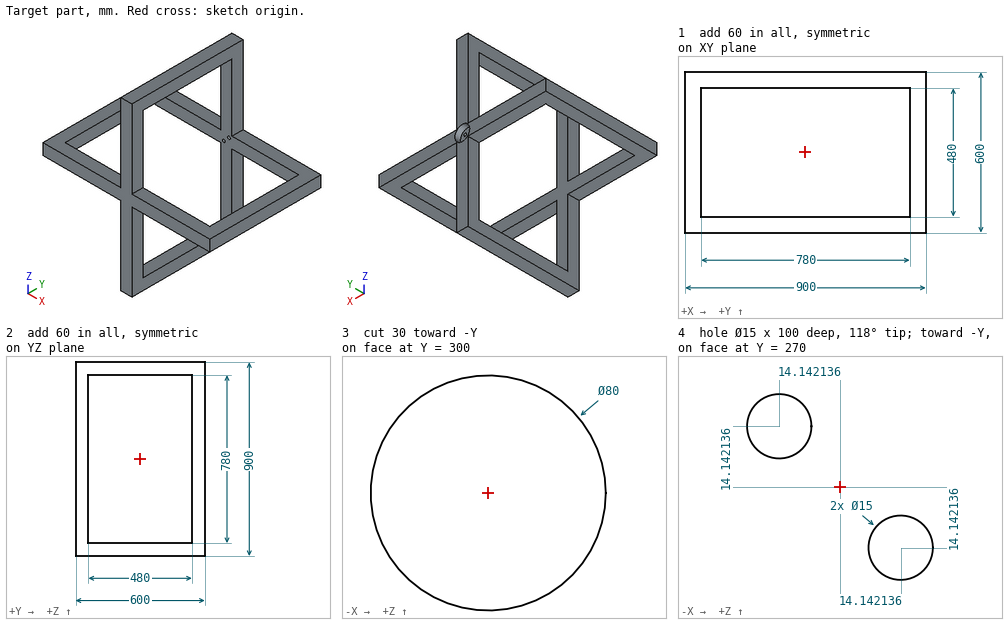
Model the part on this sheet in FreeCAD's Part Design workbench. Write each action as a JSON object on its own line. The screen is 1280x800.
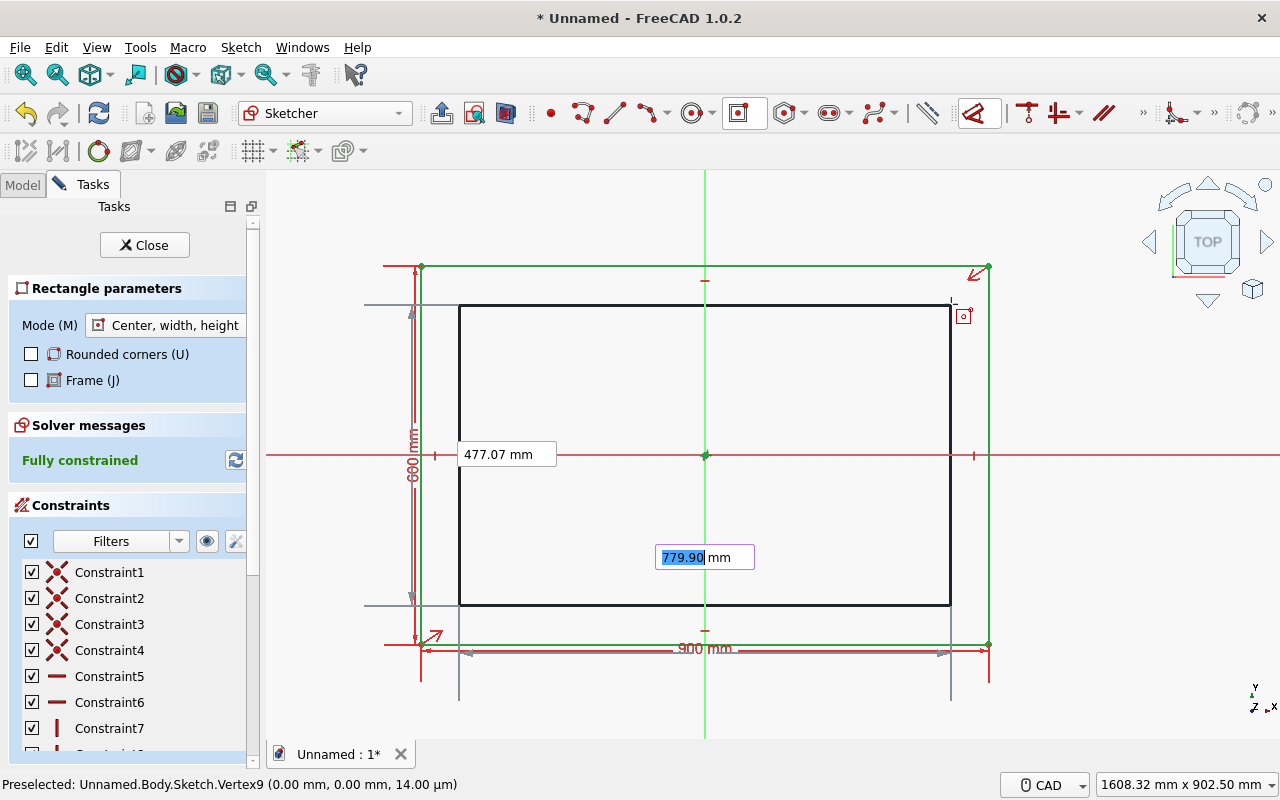
{"action": "type", "text": "780"}
{"action": "key", "text": "Tab"}
{"action": "type", "text": "480"}
{"action": "key", "text": "Return"}
{"action": "key", "text": "Escape"}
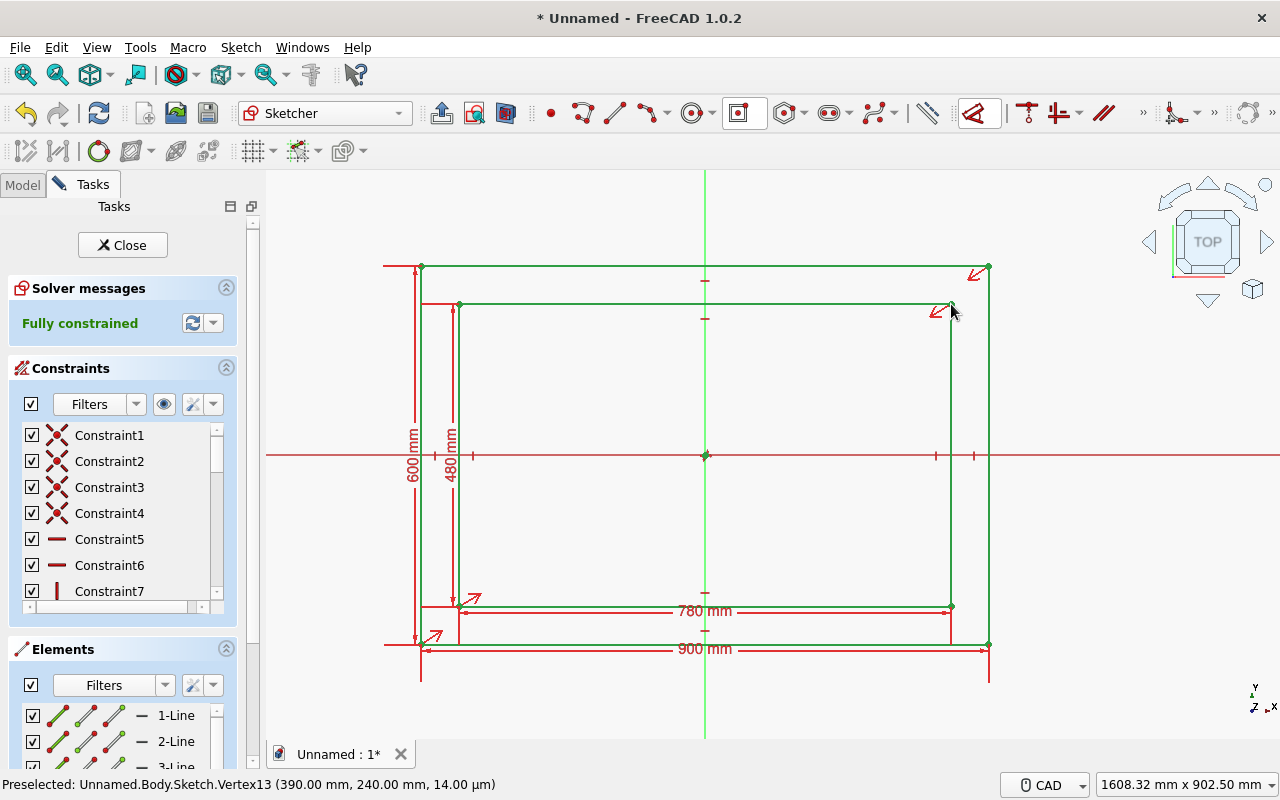
{"action": "left_click", "coordinate": [123, 245]}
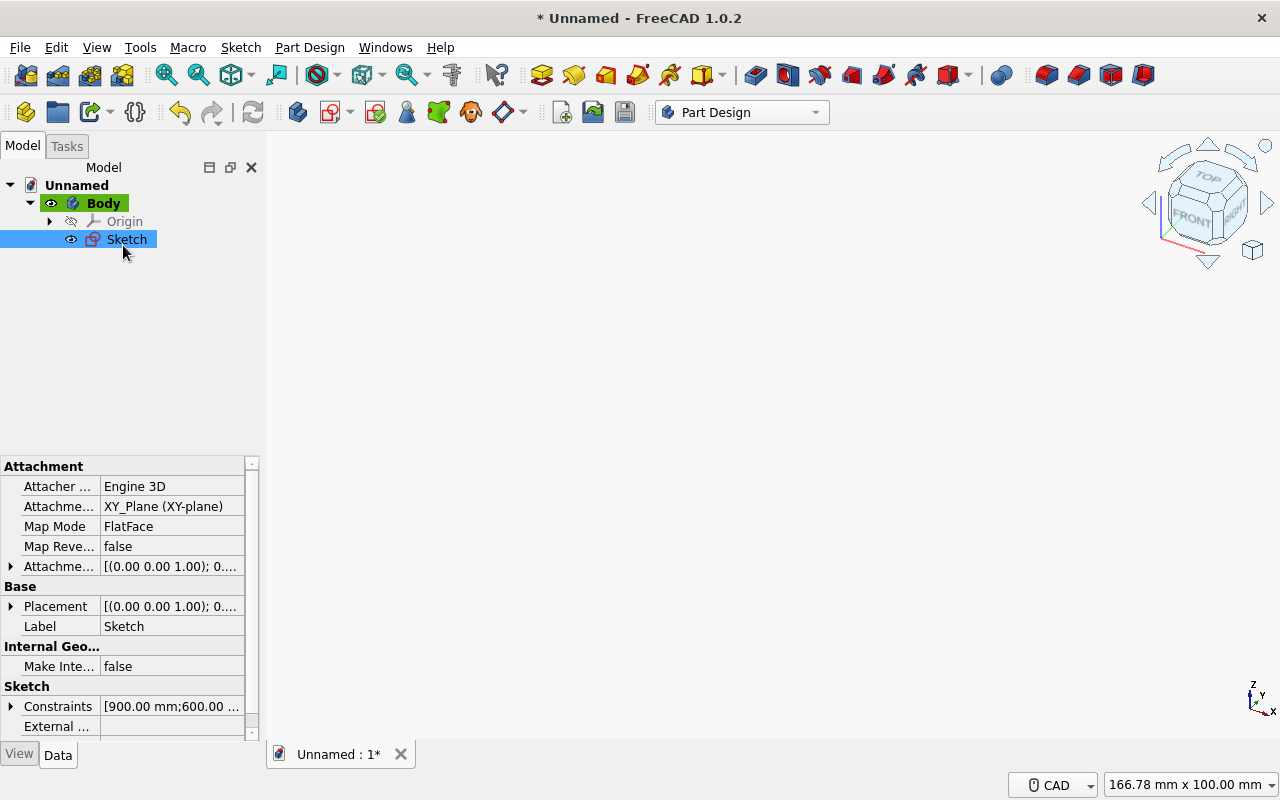
{"action": "left_click", "coordinate": [542, 76]}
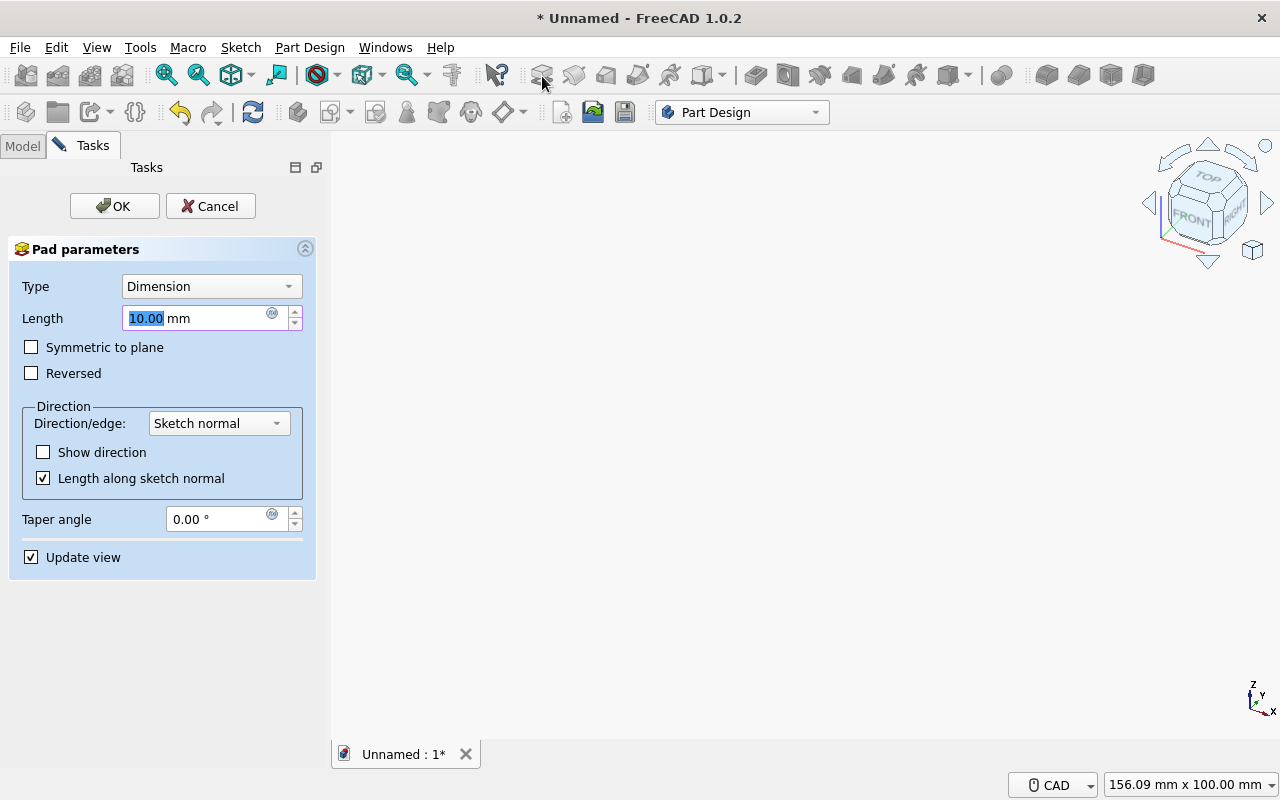
{"action": "type", "text": "60"}
{"action": "key", "text": "Tab"}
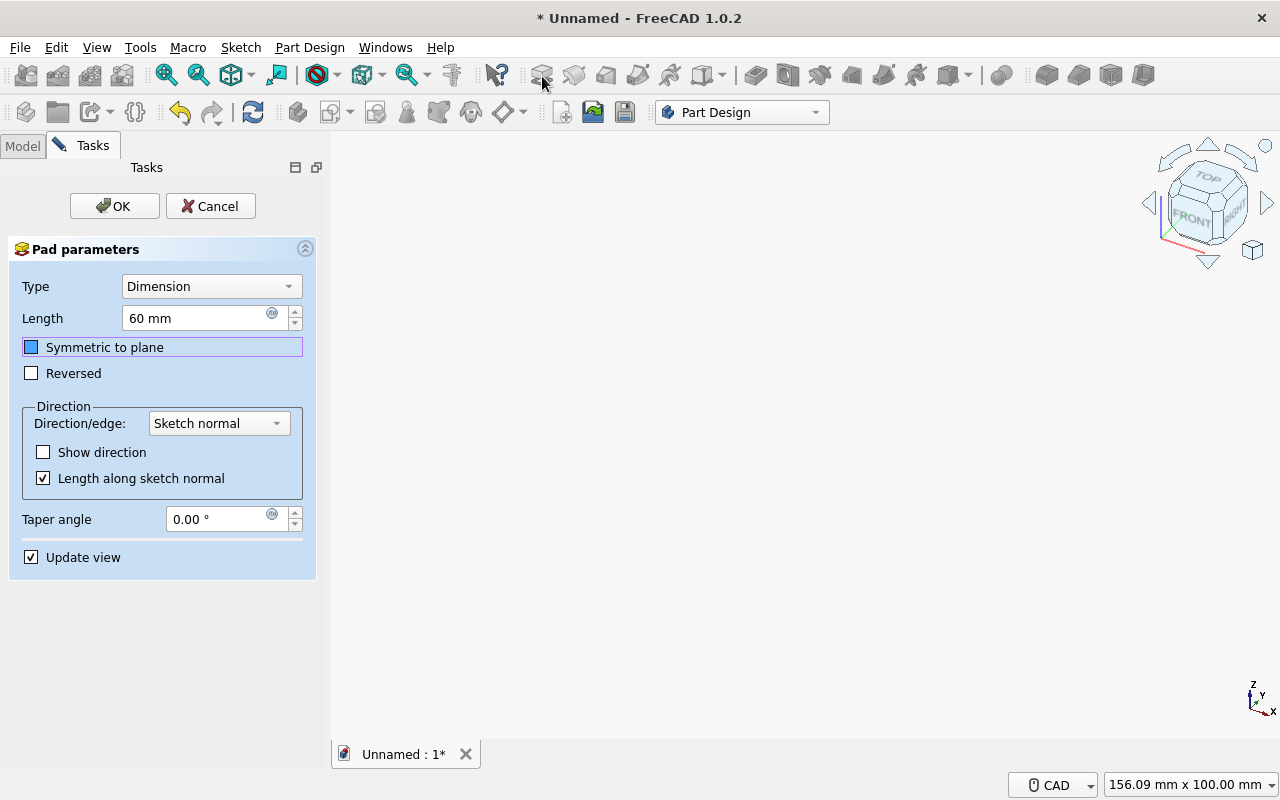
{"action": "left_click", "coordinate": [30, 347]}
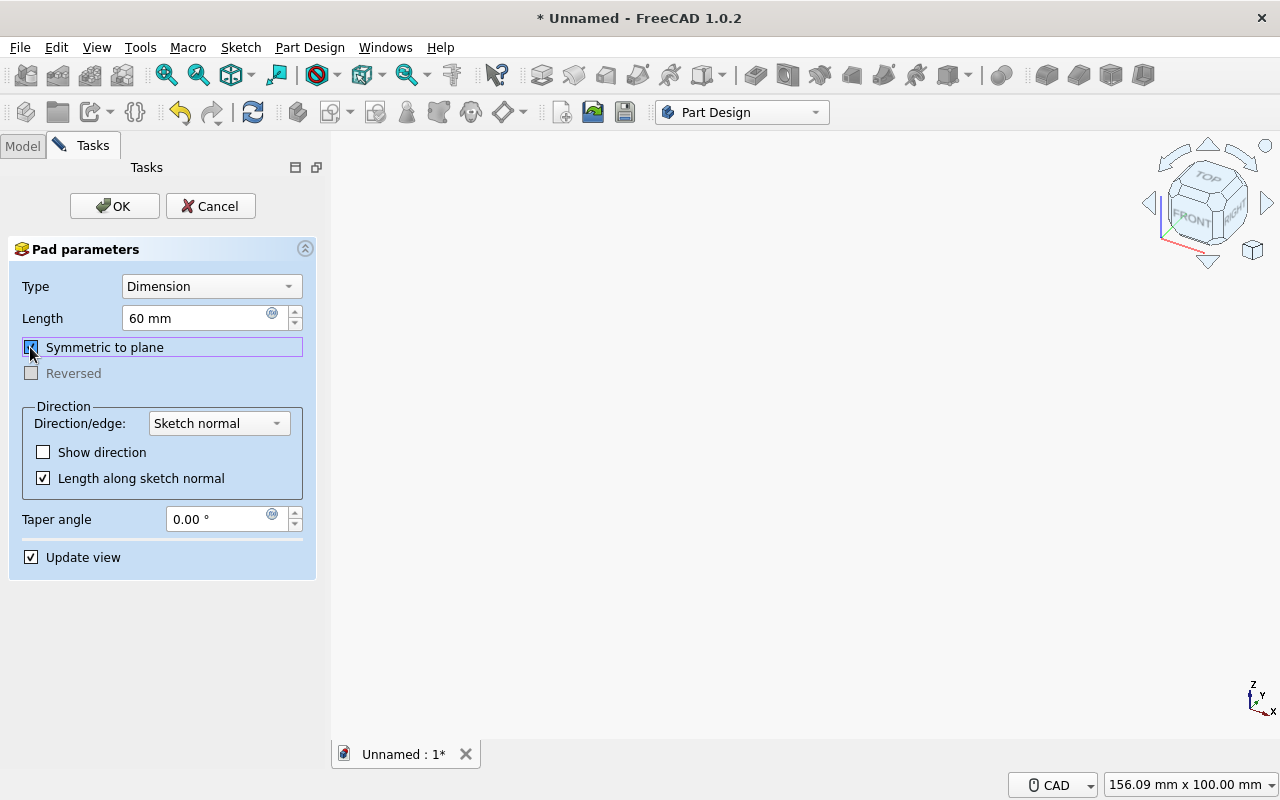
{"action": "left_click", "coordinate": [115, 206]}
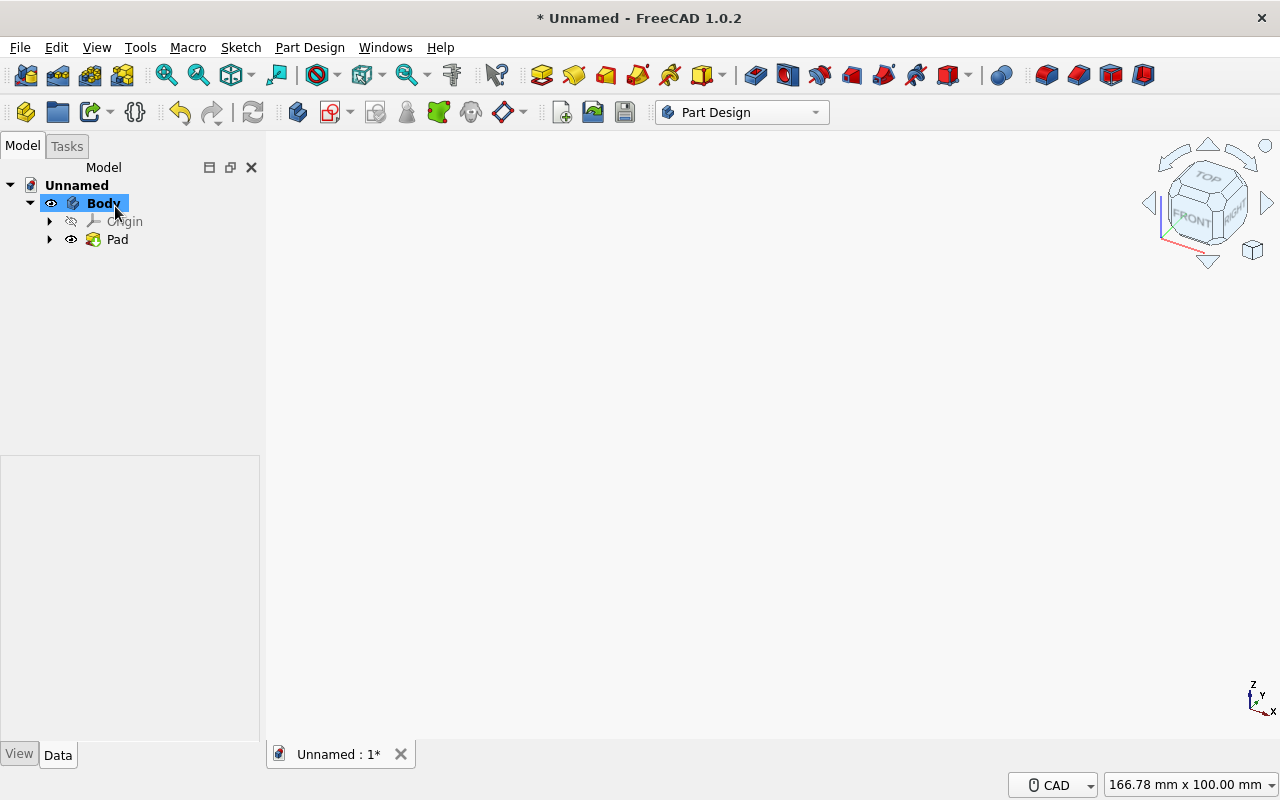
{"action": "left_click", "coordinate": [168, 76]}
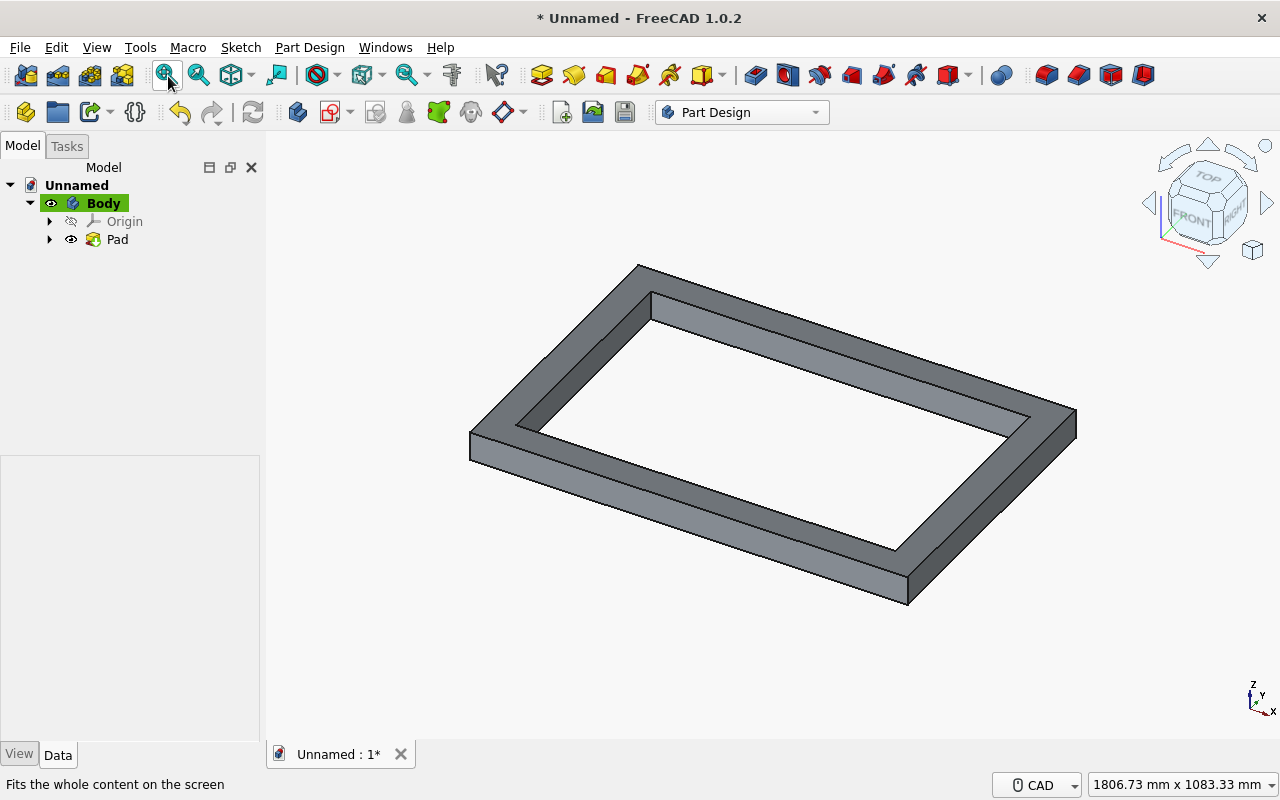
{"action": "left_click", "coordinate": [330, 112]}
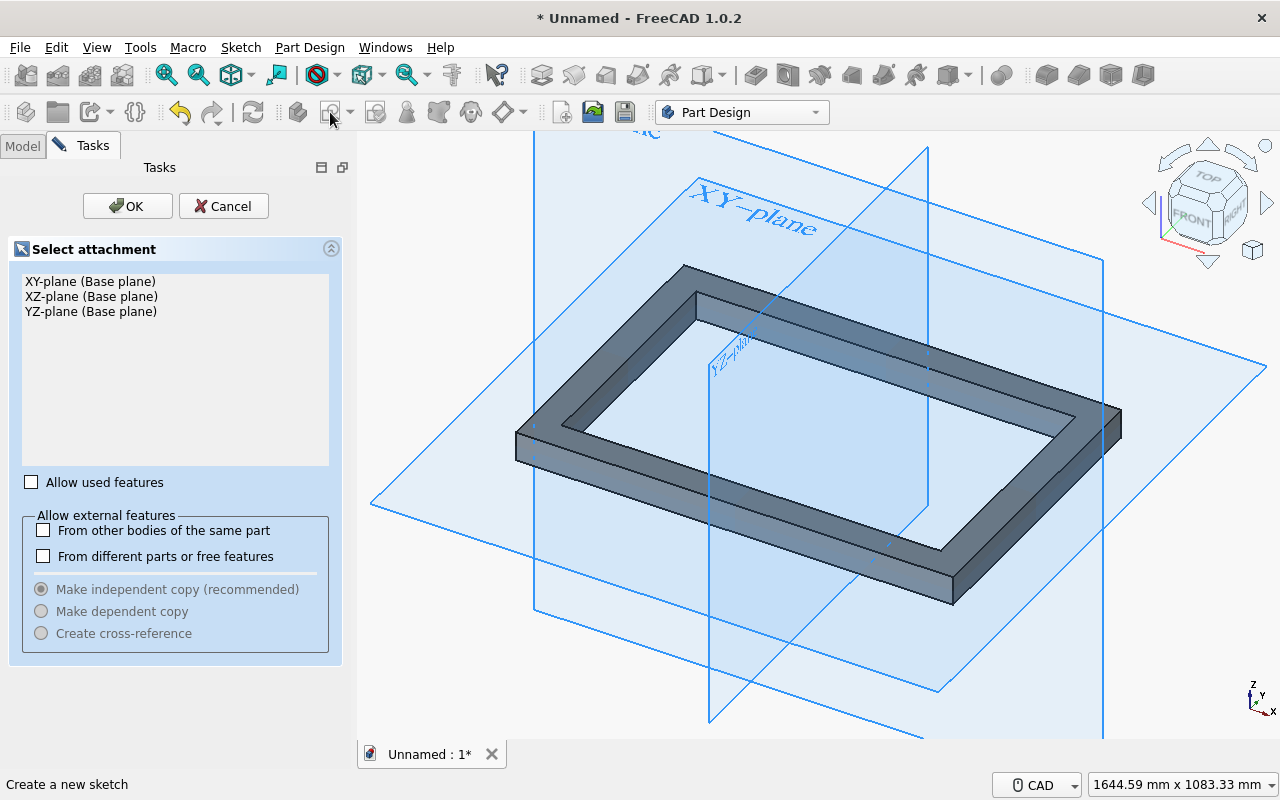
{"action": "left_click", "coordinate": [82, 312]}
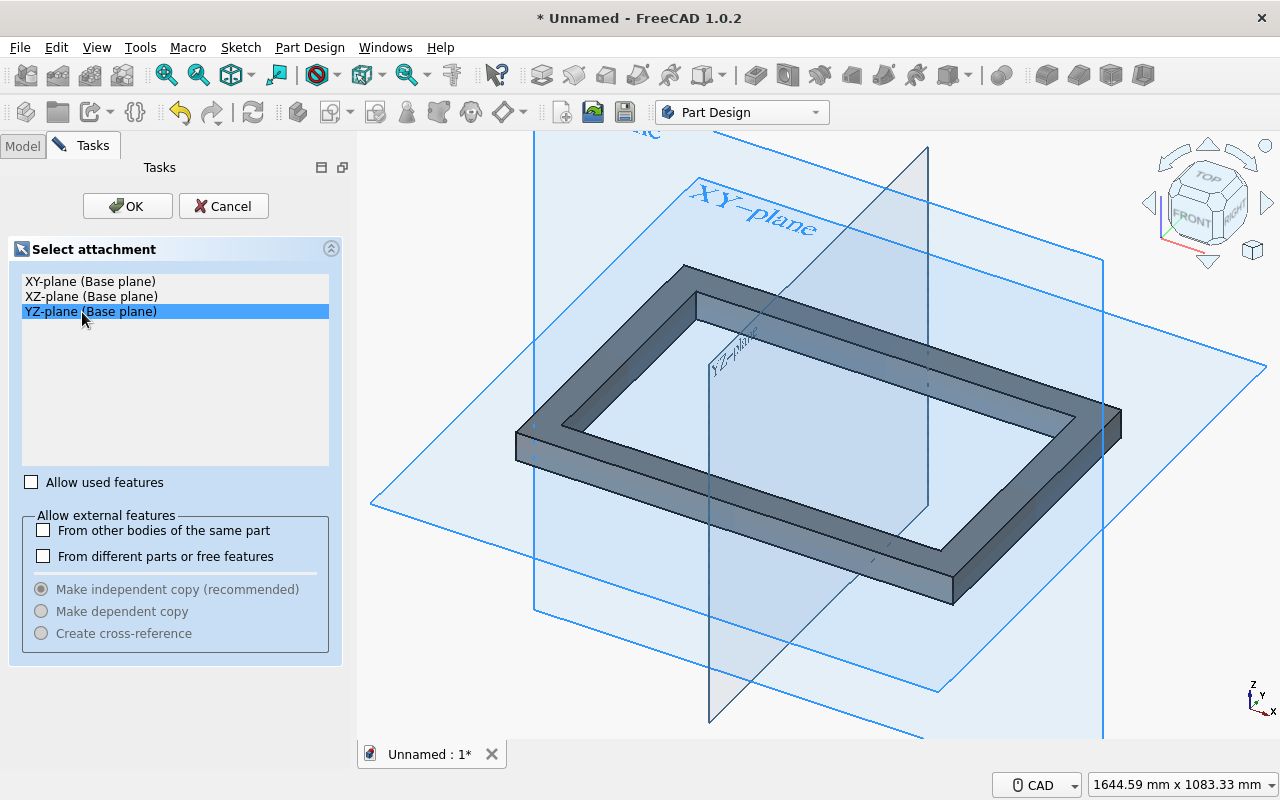
{"action": "left_click", "coordinate": [128, 206]}